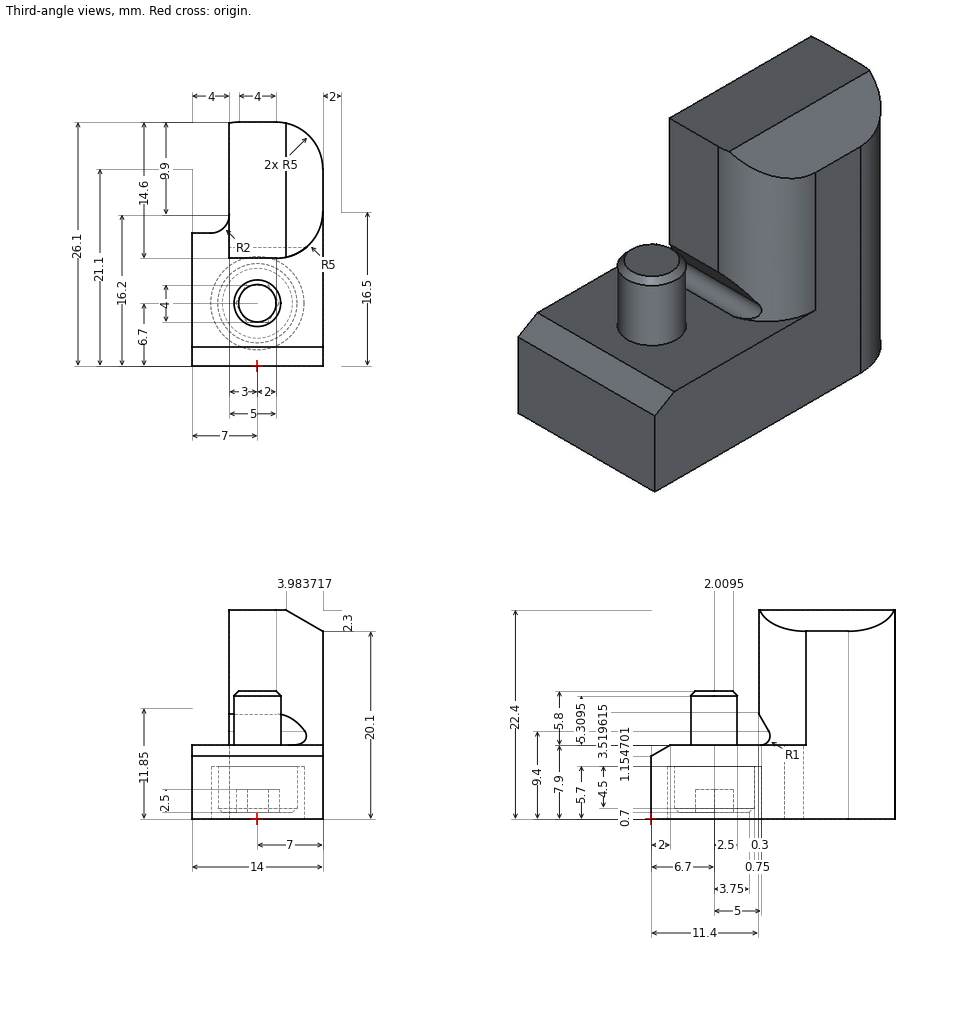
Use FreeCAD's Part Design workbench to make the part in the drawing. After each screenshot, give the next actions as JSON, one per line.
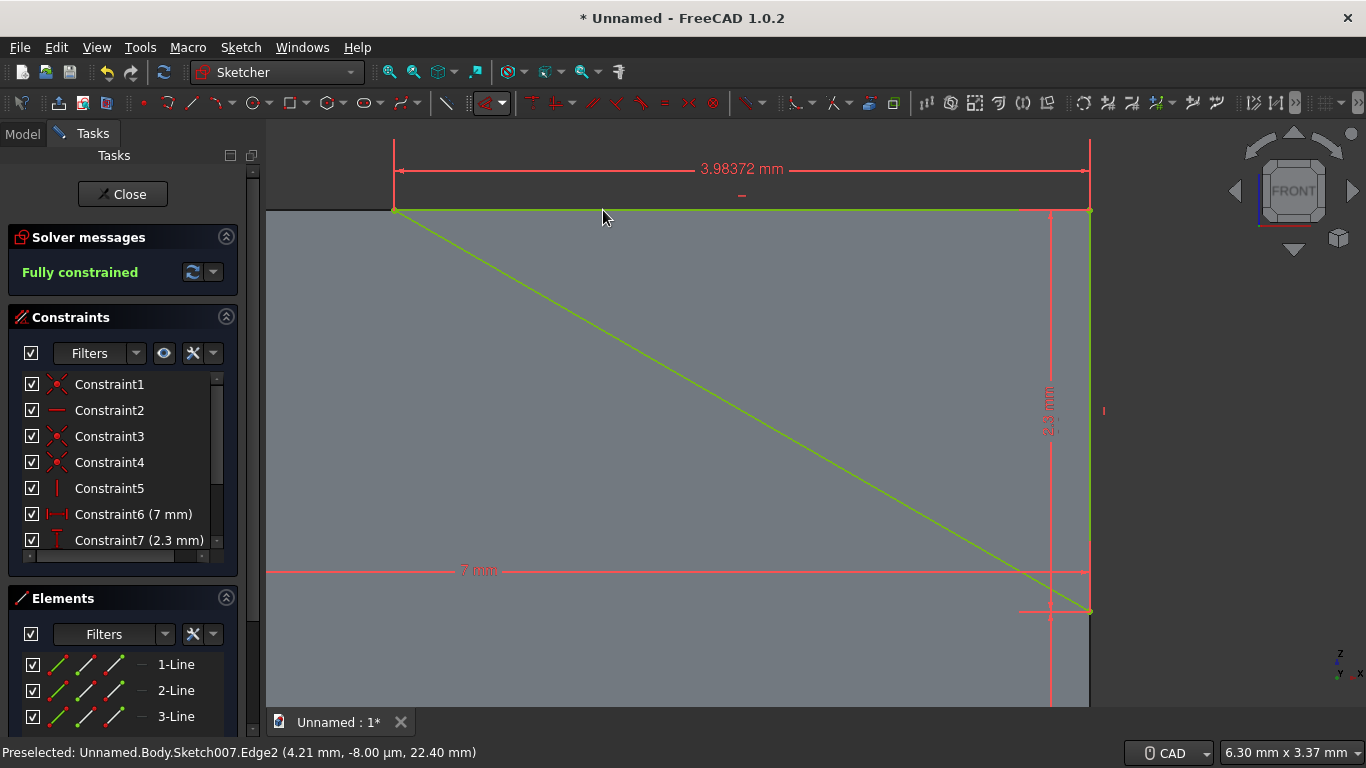
{"action": "left_click", "coordinate": [123, 194]}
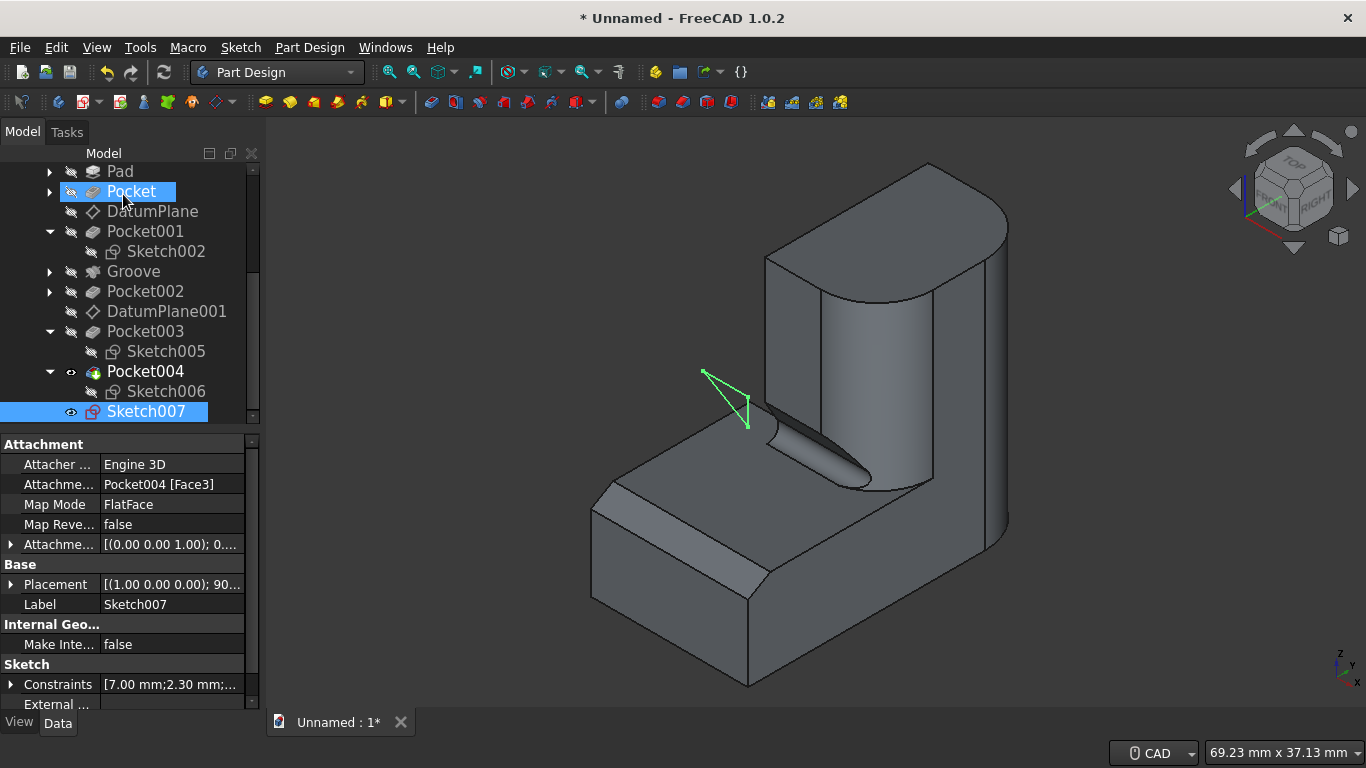
{"action": "left_click", "coordinate": [432, 102]}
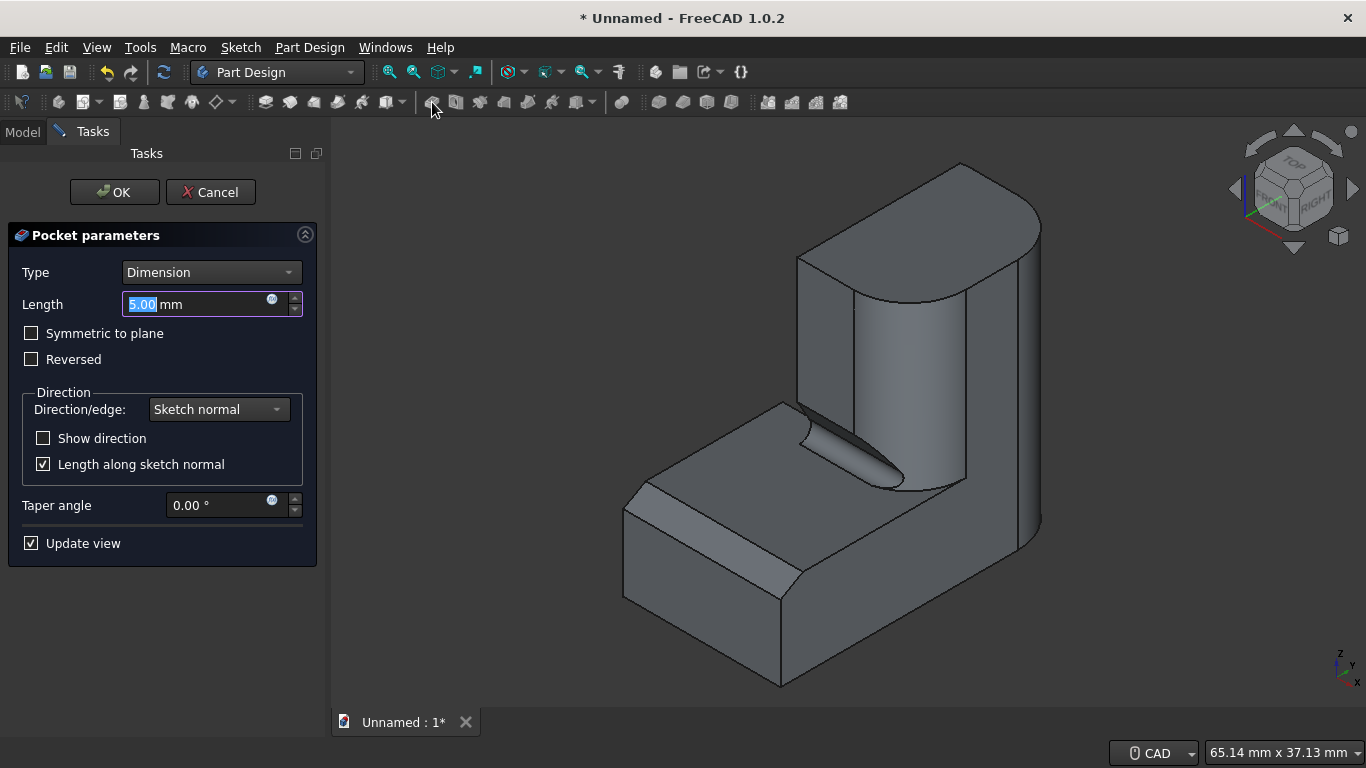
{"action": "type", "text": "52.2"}
{"action": "key", "text": "Tab"}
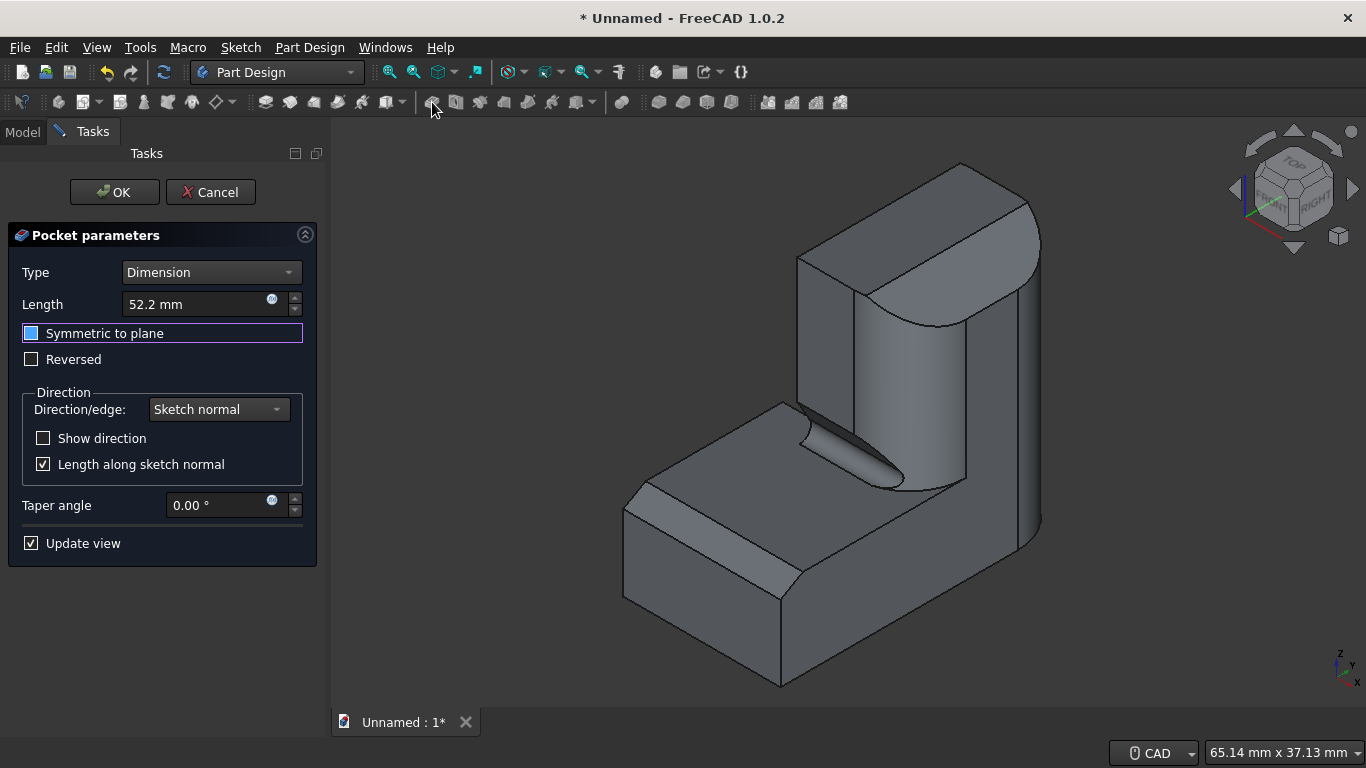
{"action": "left_click", "coordinate": [30, 333]}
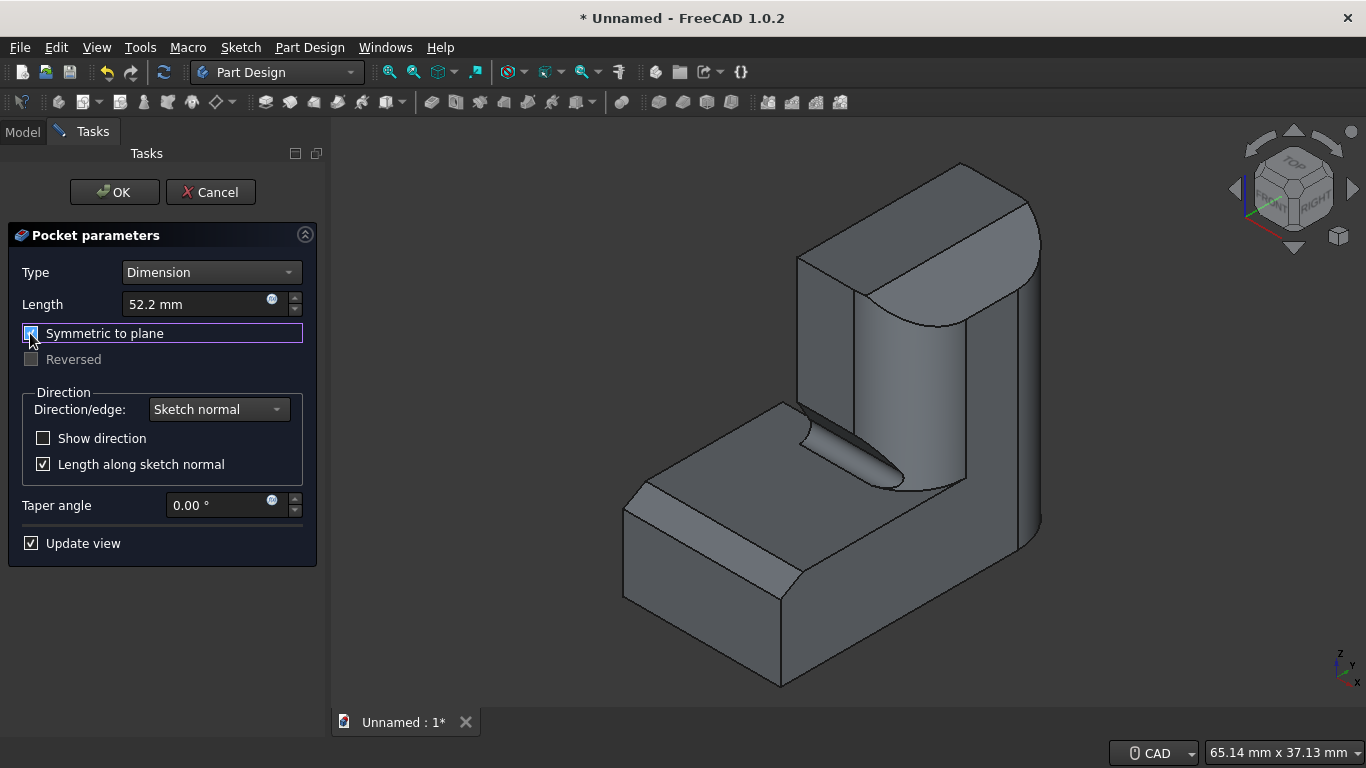
{"action": "left_click", "coordinate": [115, 192]}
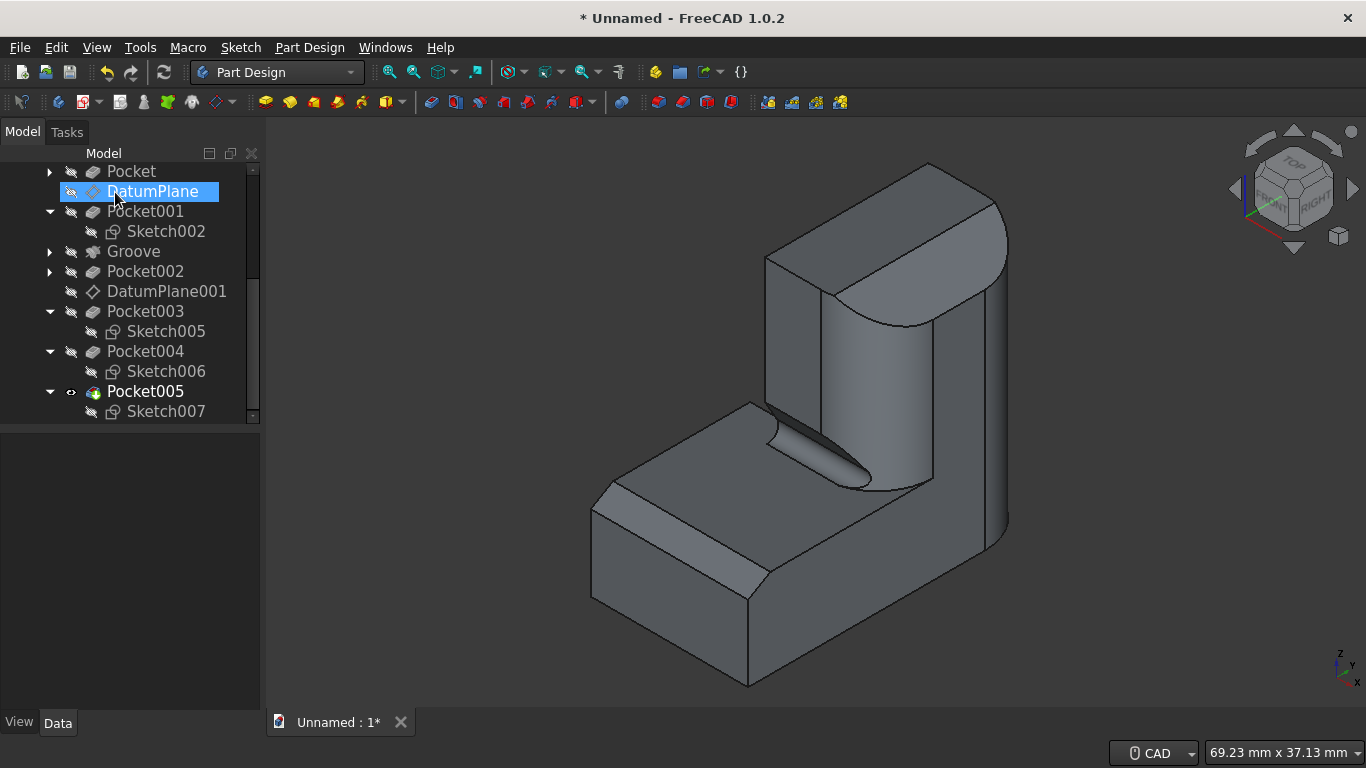
{"action": "left_click", "coordinate": [84, 102]}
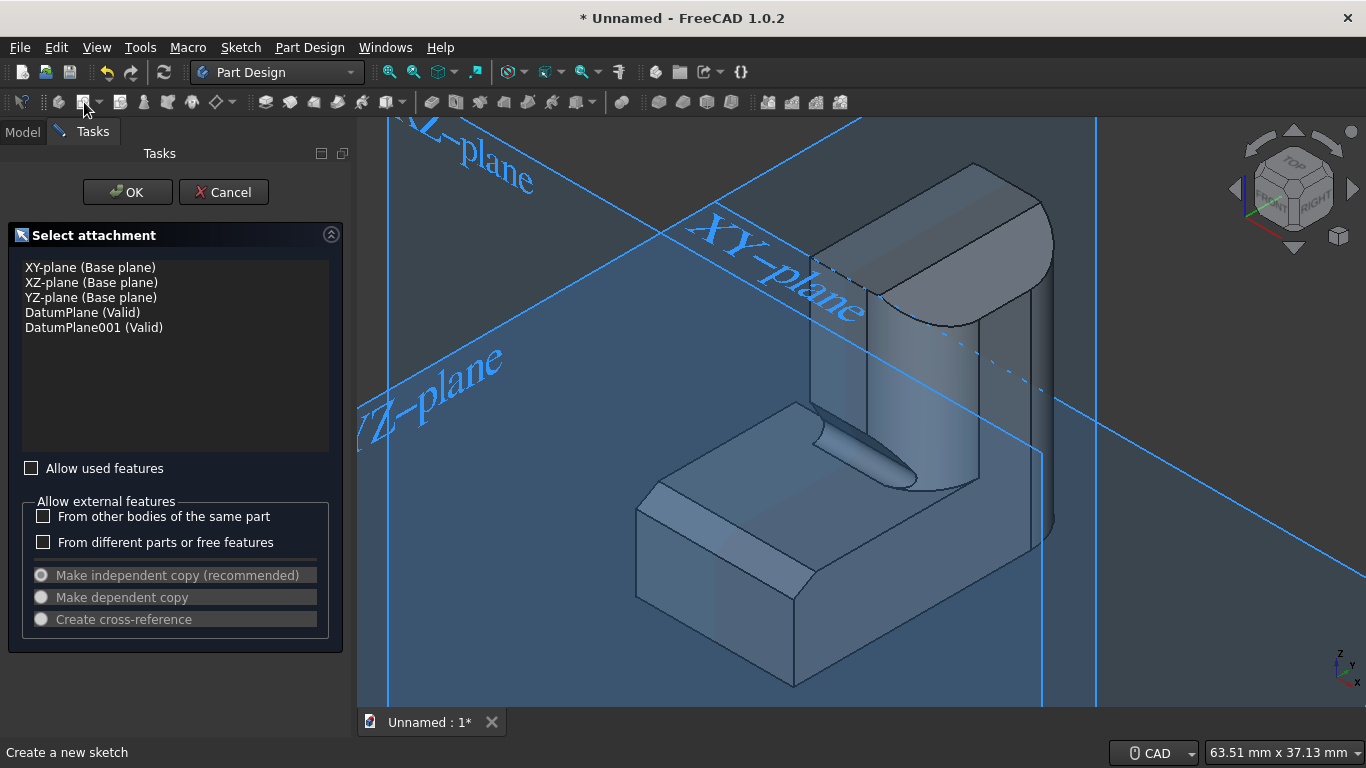
{"action": "left_click", "coordinate": [82, 298]}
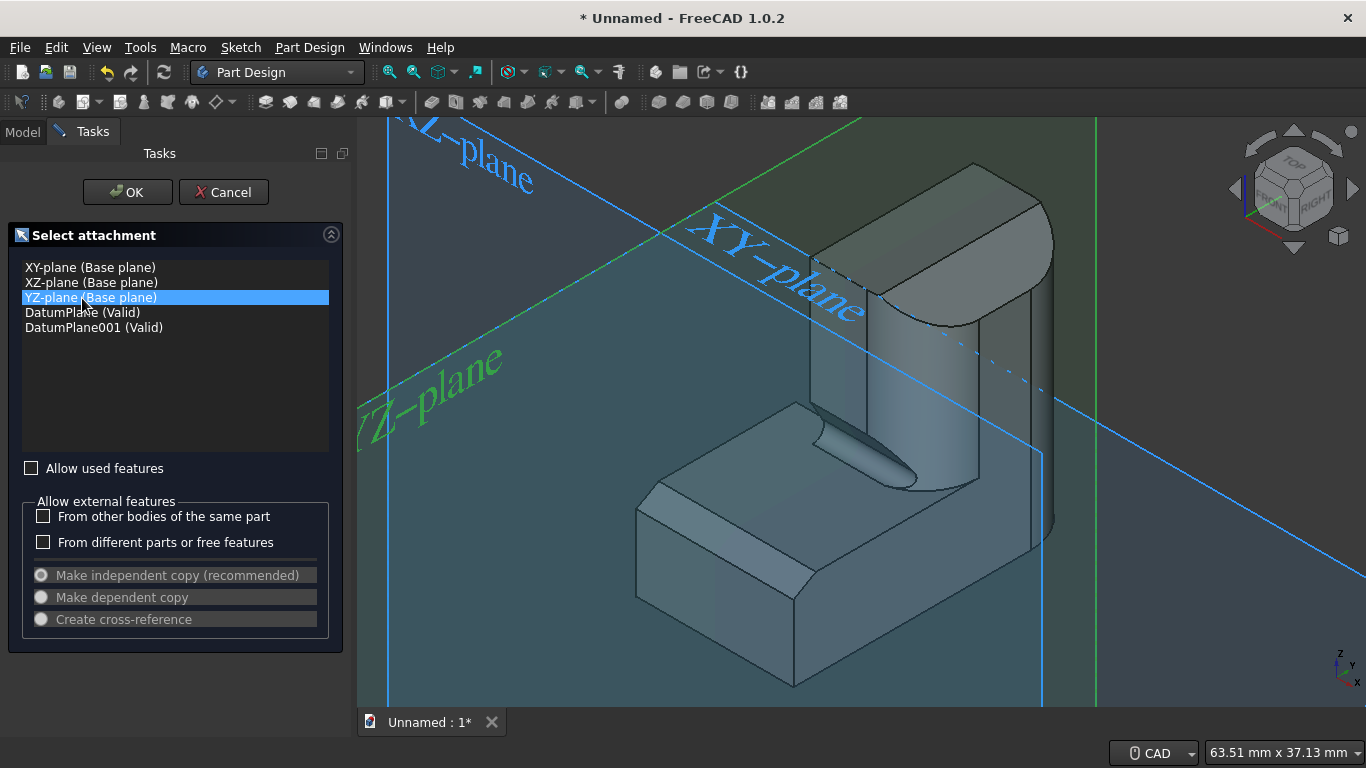
{"action": "left_click", "coordinate": [128, 192]}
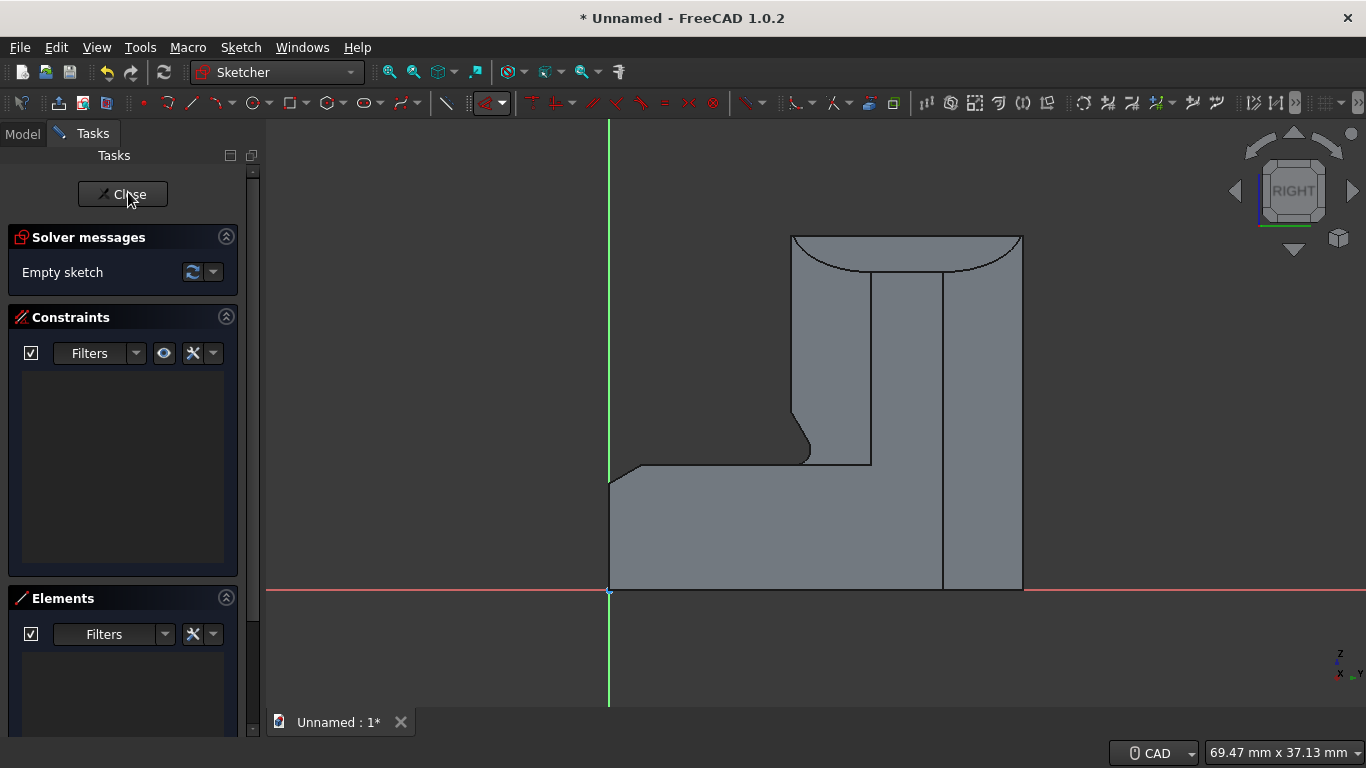
{"action": "left_click", "coordinate": [108, 104]}